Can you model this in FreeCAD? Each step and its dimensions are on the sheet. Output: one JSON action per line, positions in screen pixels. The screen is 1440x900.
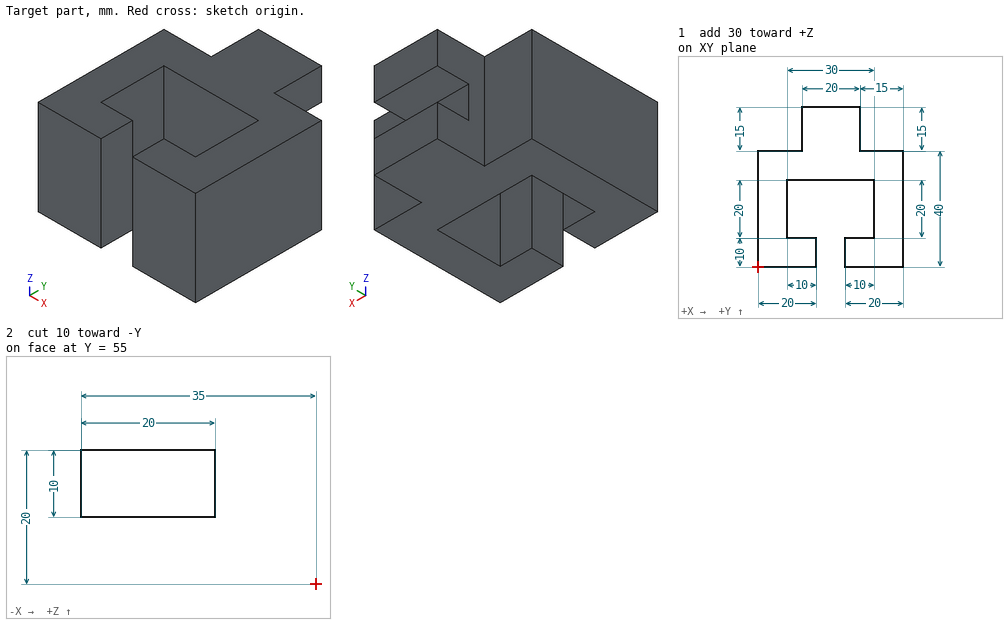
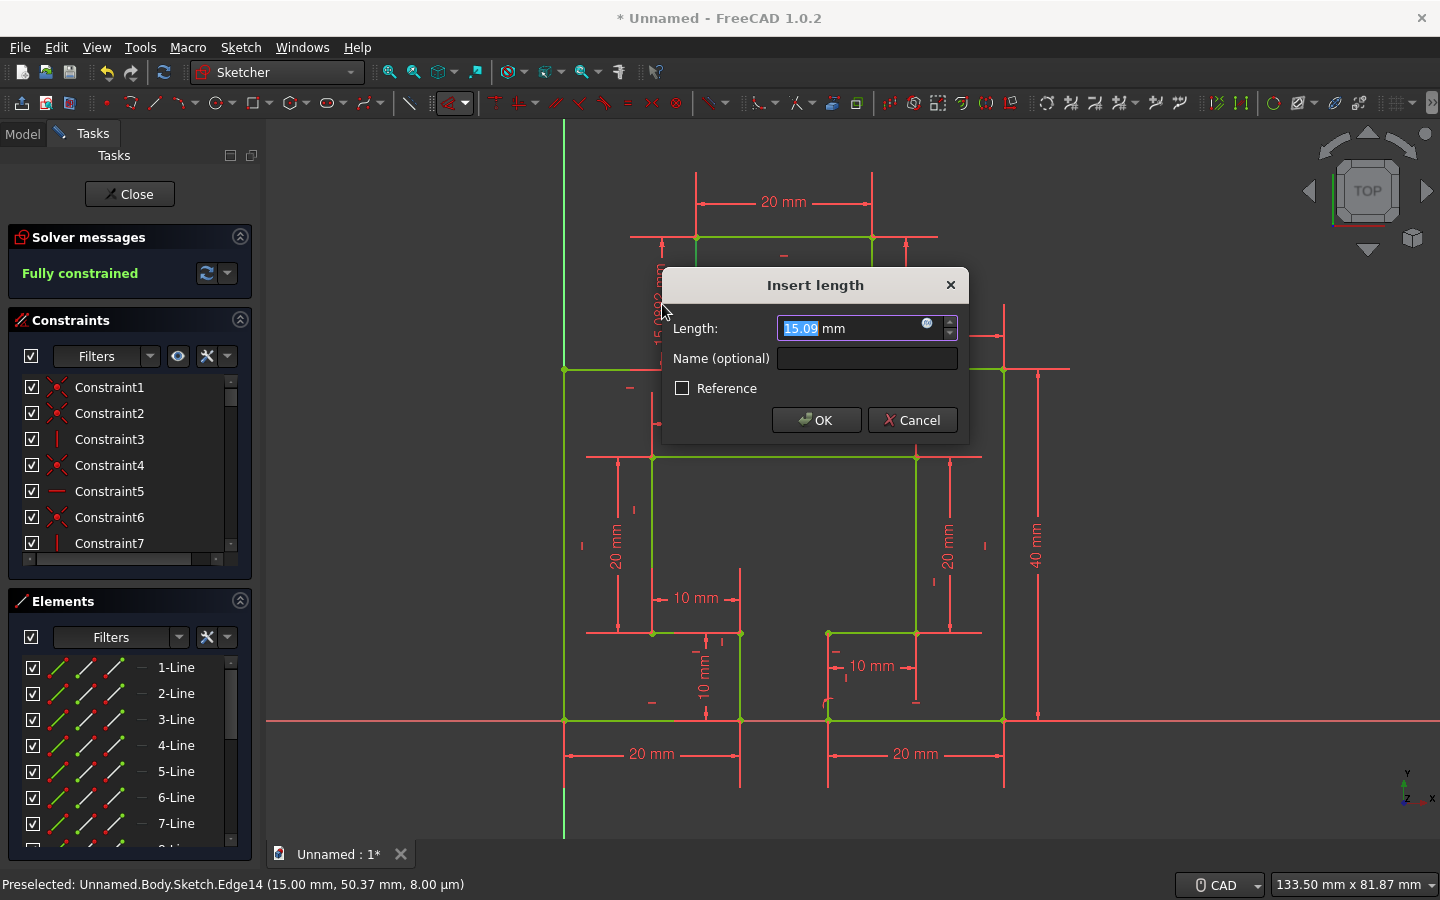
{"action": "type", "text": "15"}
{"action": "key", "text": "Return"}
{"action": "key", "text": "Escape"}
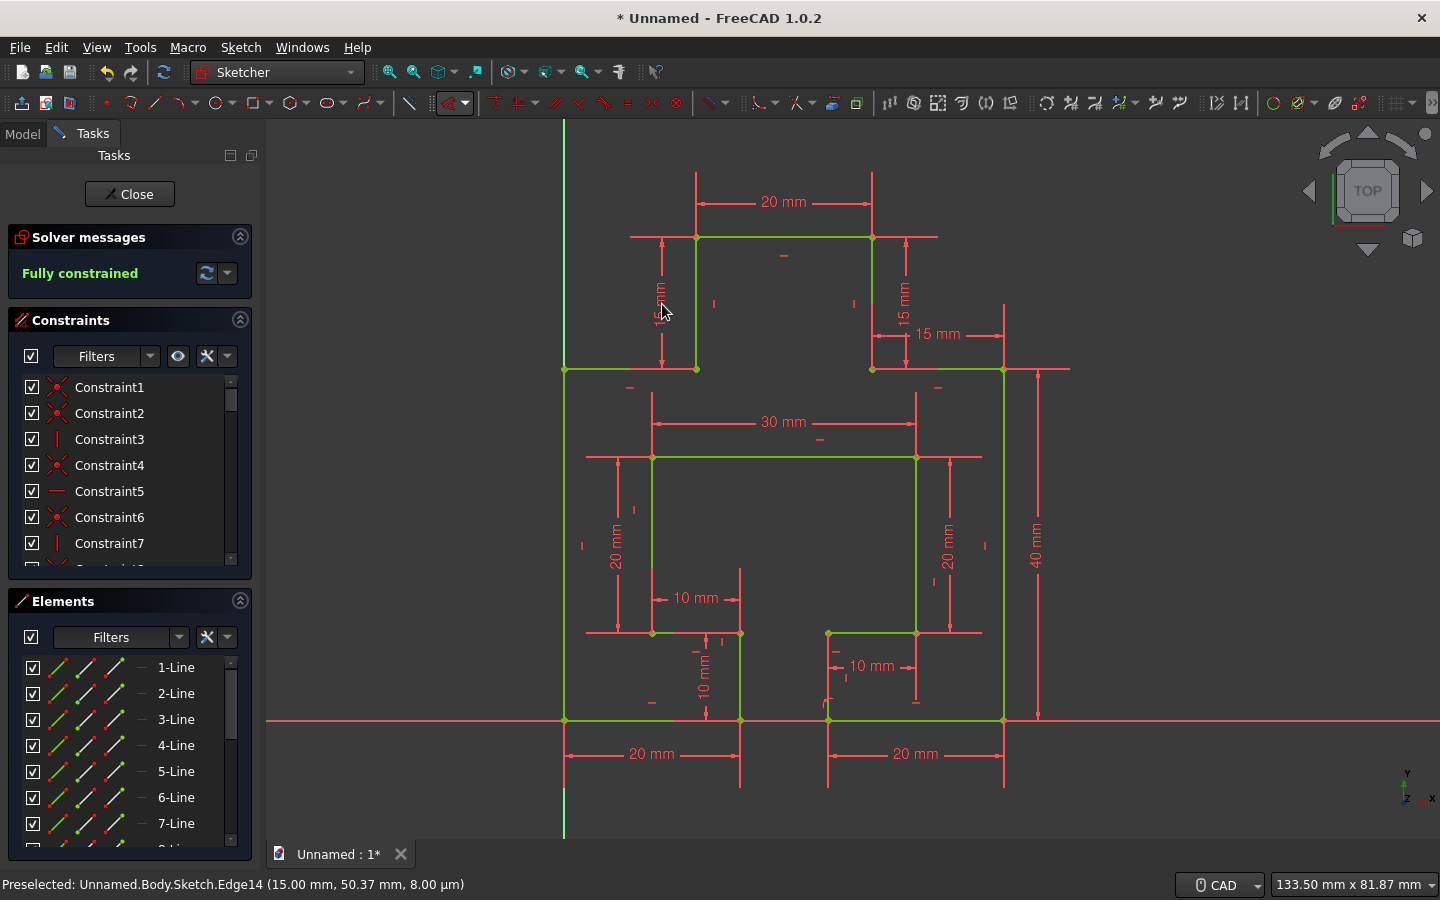
{"action": "left_click", "coordinate": [130, 194]}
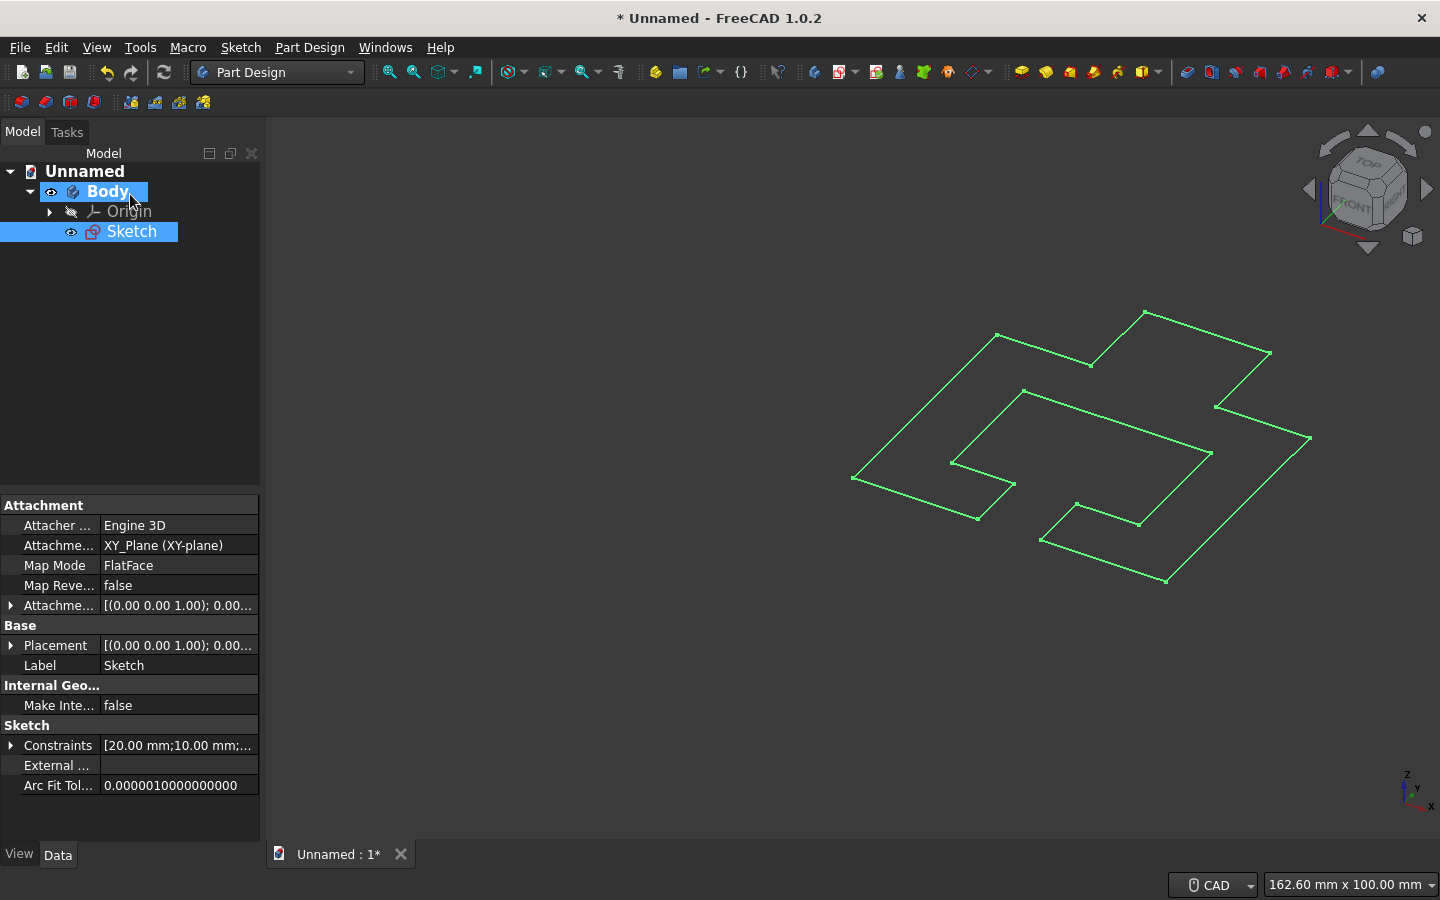
{"action": "left_click", "coordinate": [1022, 72]}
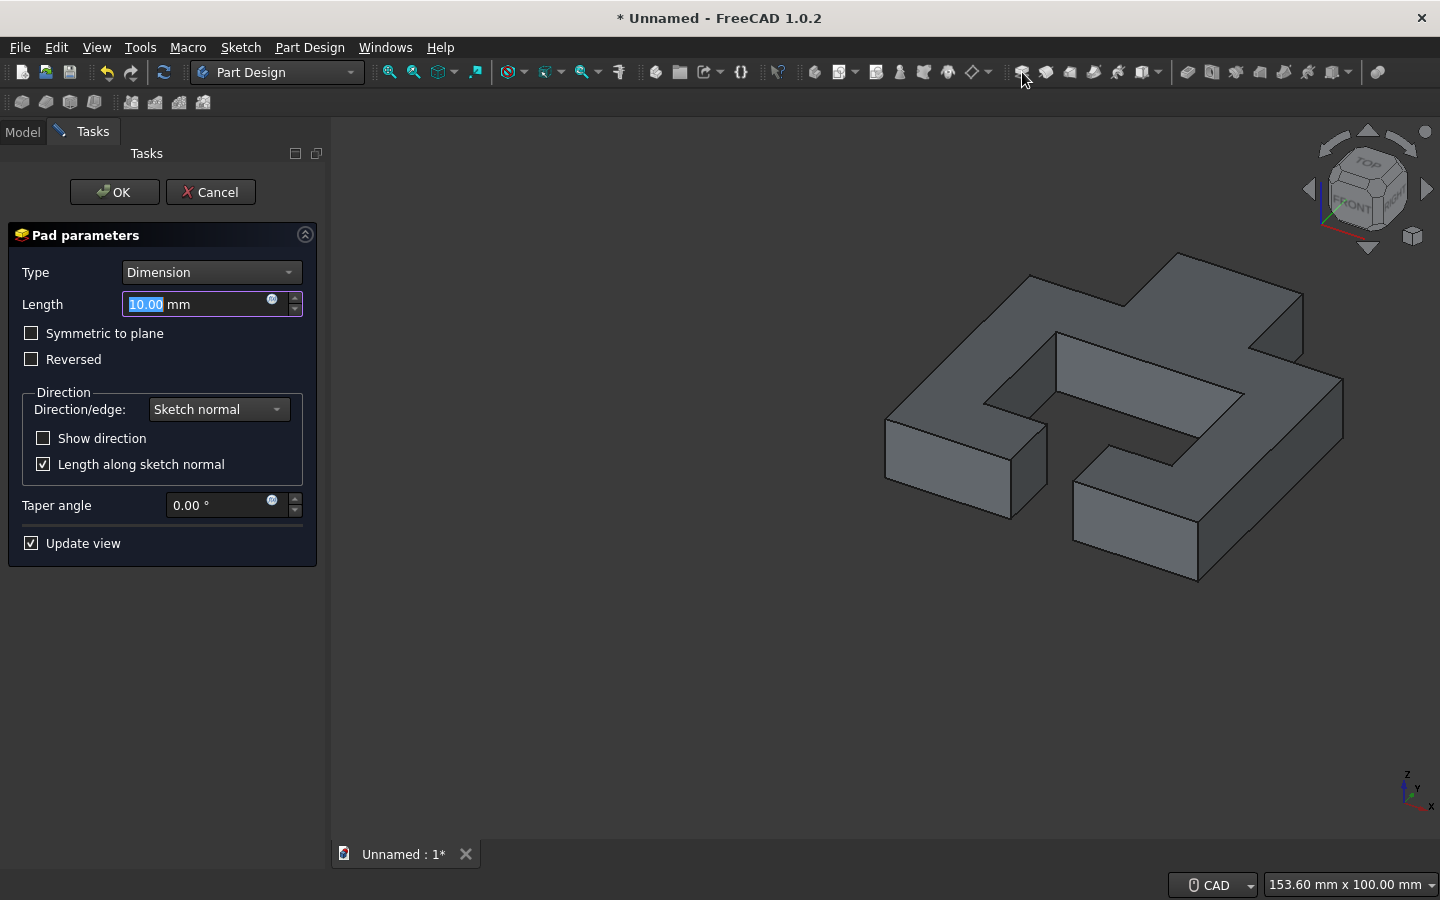
{"action": "type", "text": "30"}
{"action": "key", "text": "Tab"}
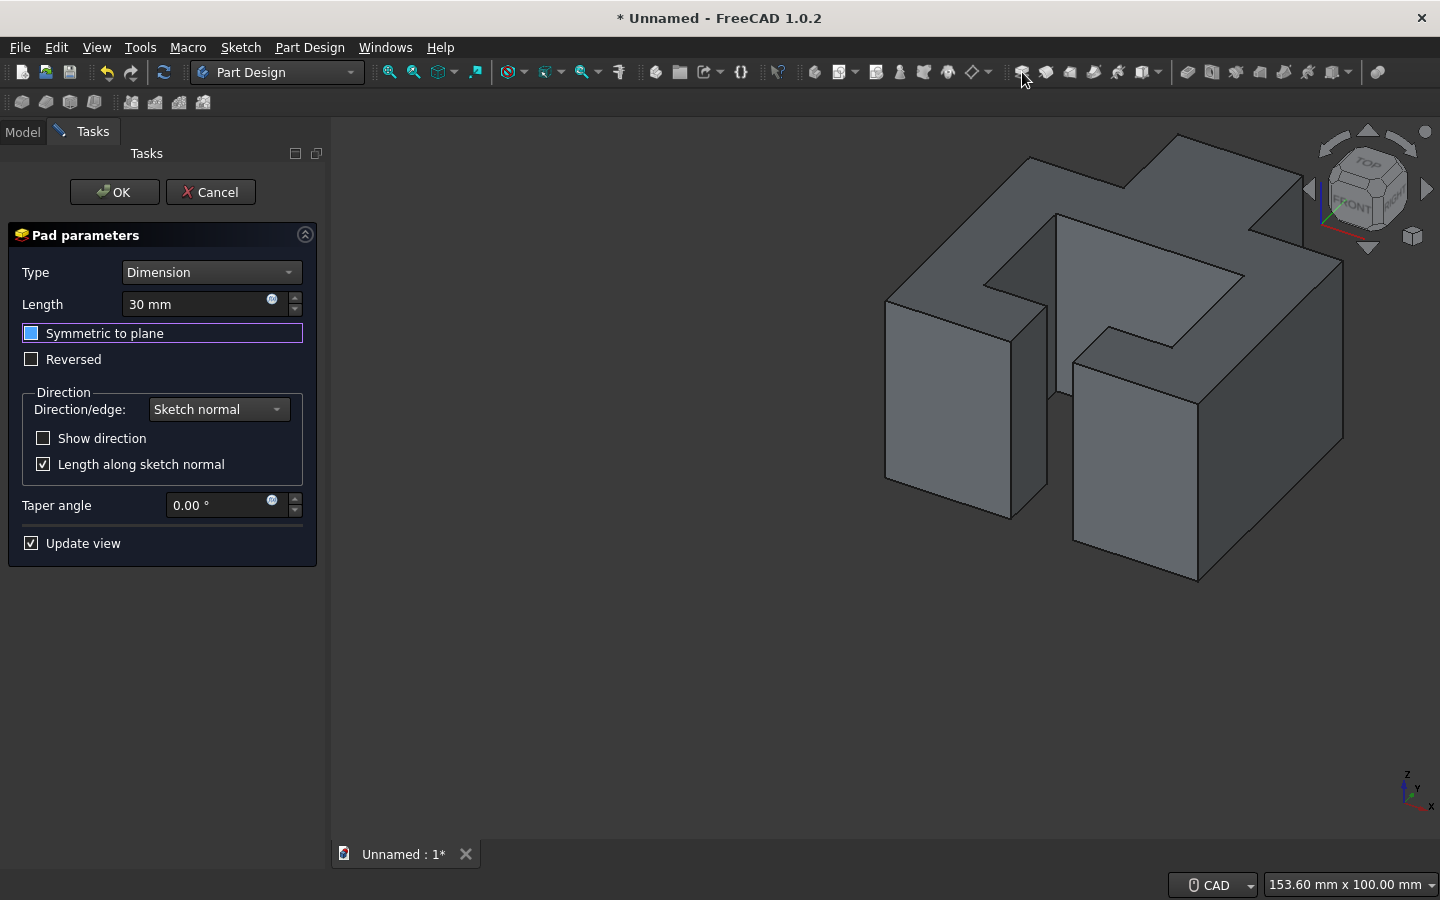
{"action": "left_click", "coordinate": [115, 192]}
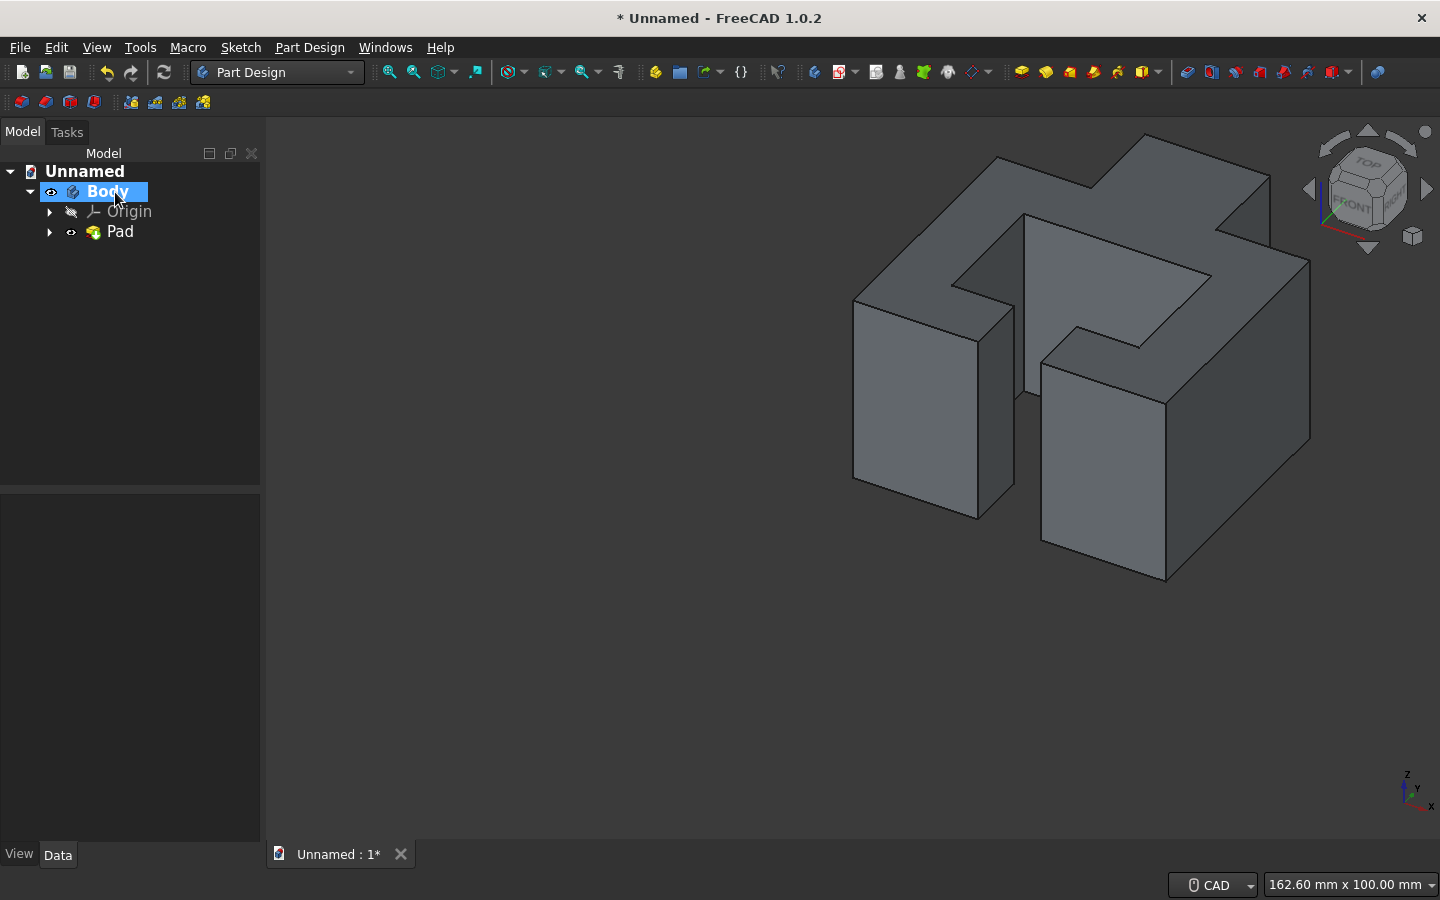
{"action": "left_click", "coordinate": [390, 72]}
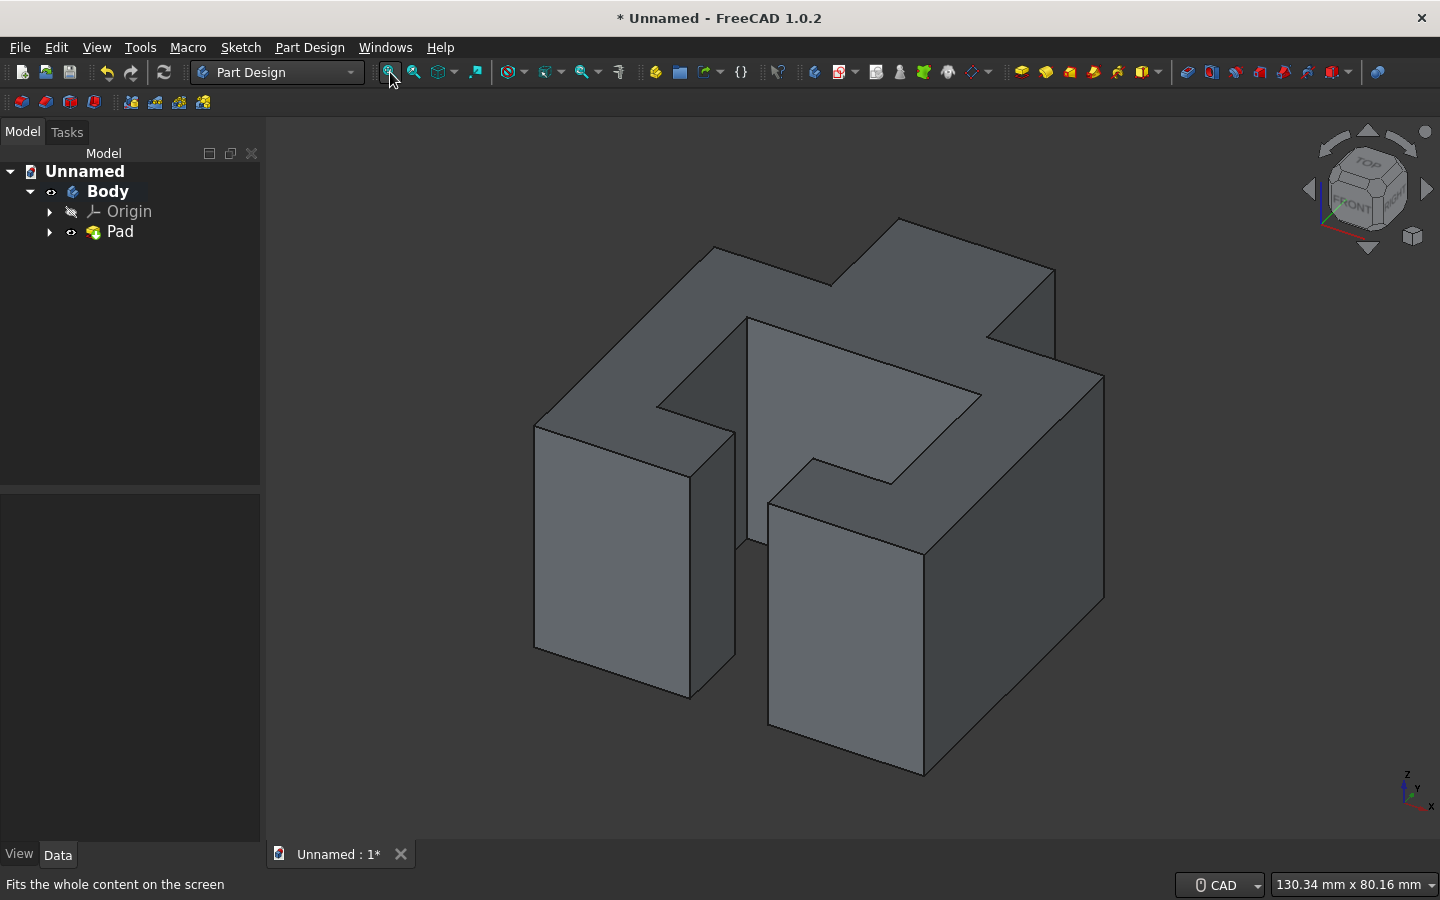
{"action": "key", "text": "4"}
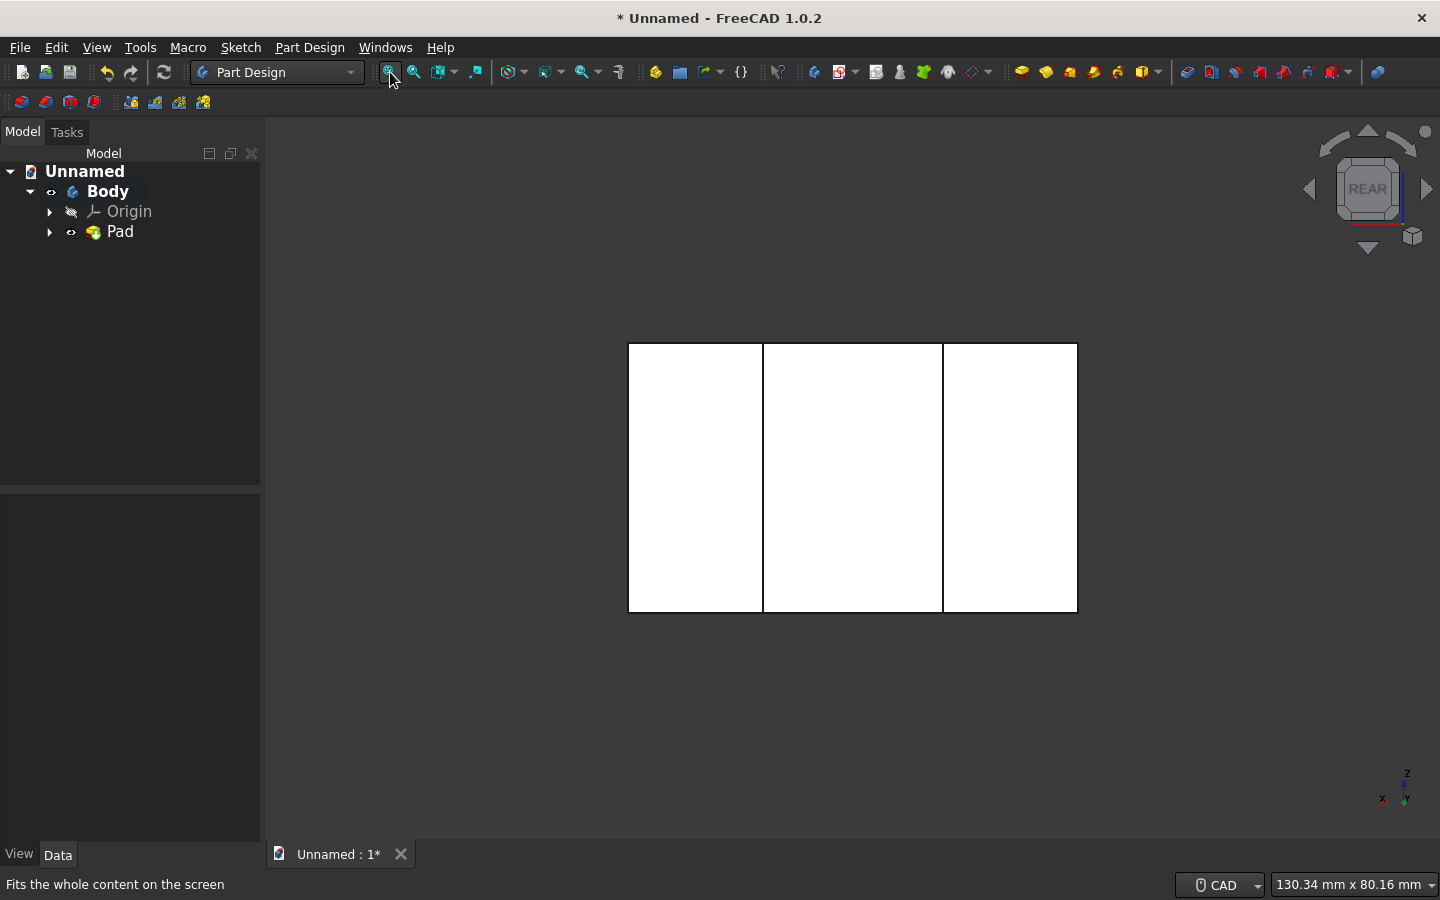
{"action": "left_click", "coordinate": [390, 72]}